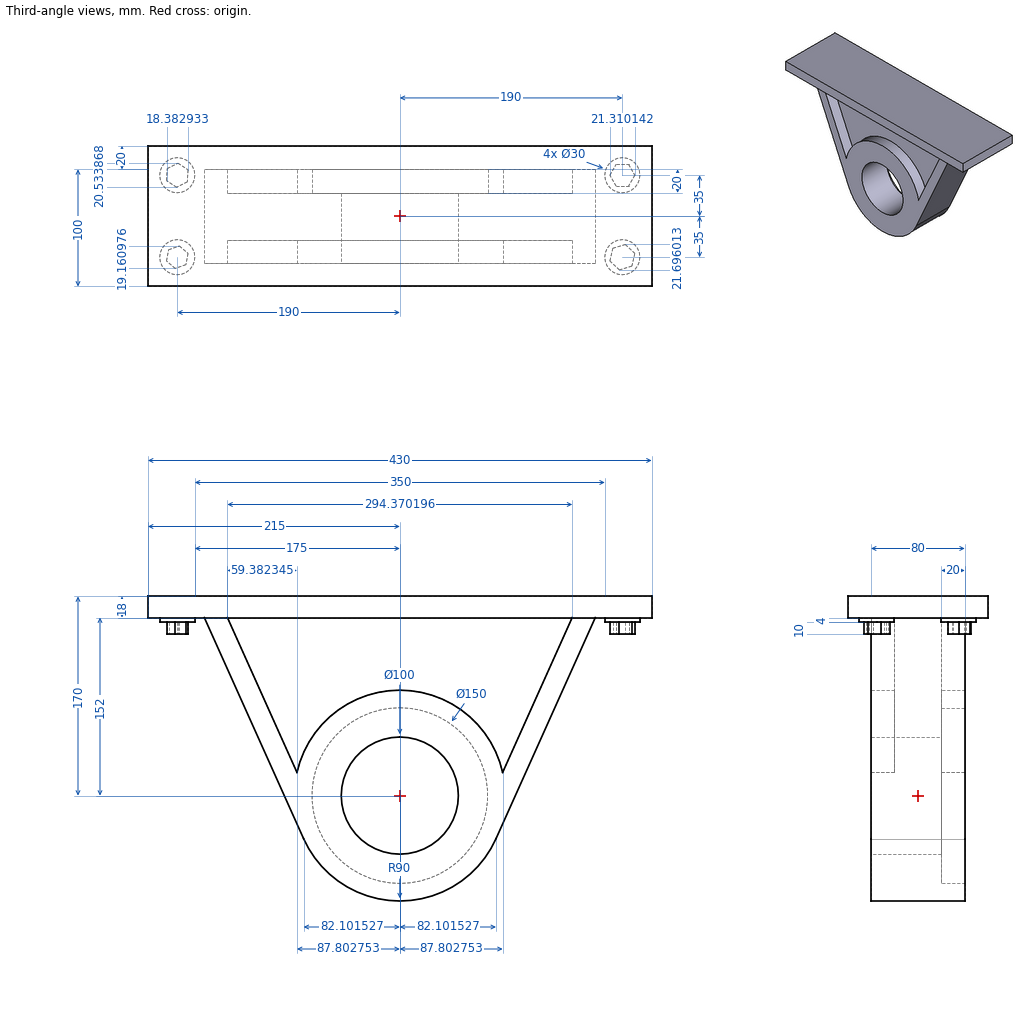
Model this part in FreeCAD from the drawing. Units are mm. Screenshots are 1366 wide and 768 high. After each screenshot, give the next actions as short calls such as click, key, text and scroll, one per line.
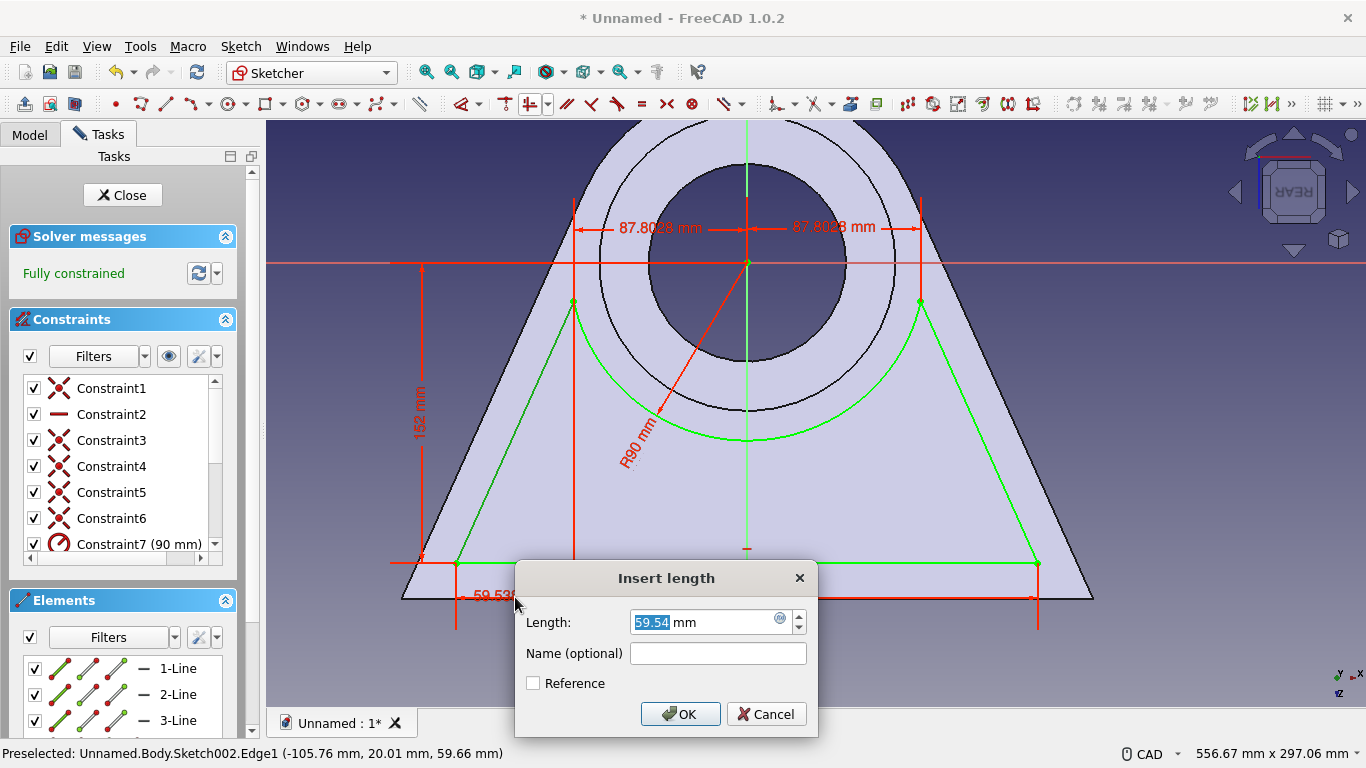
text(59.382345)
key(Return)
key(Escape)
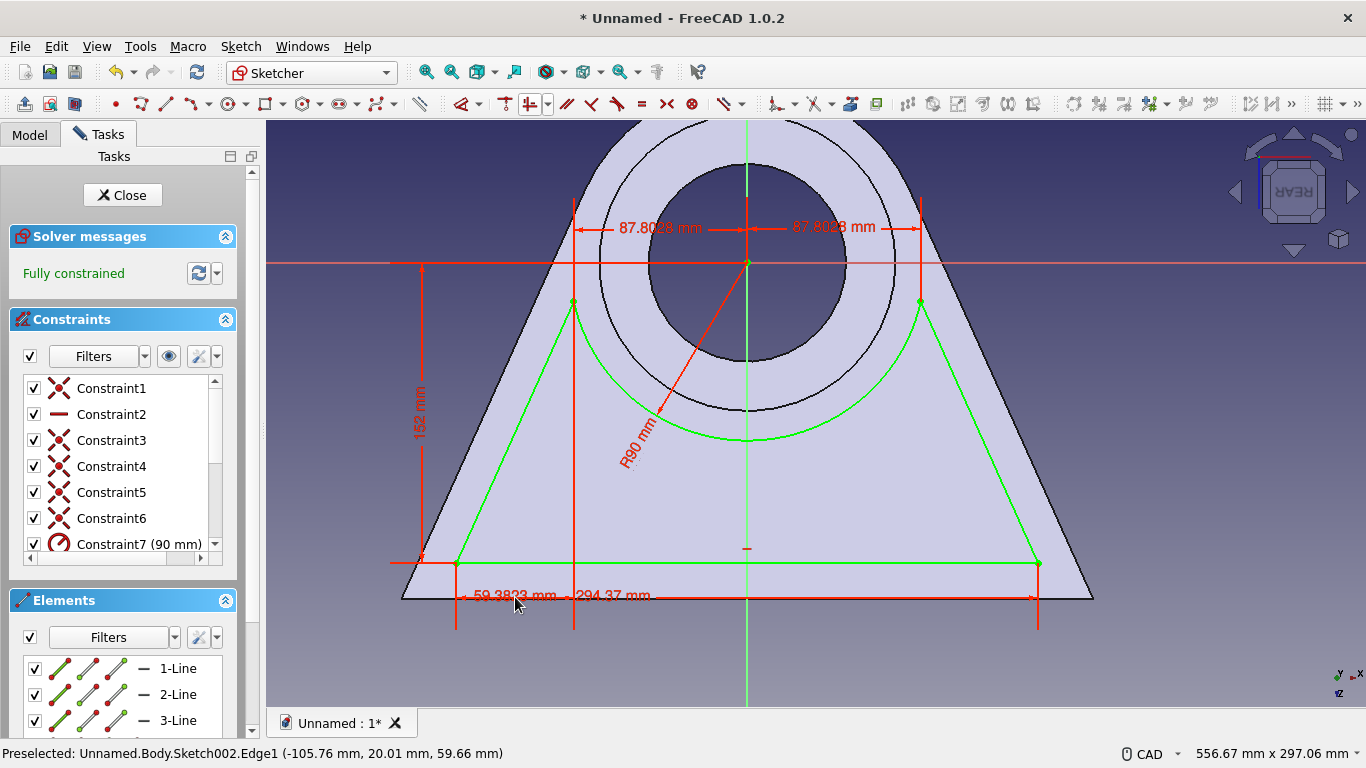
click(123, 195)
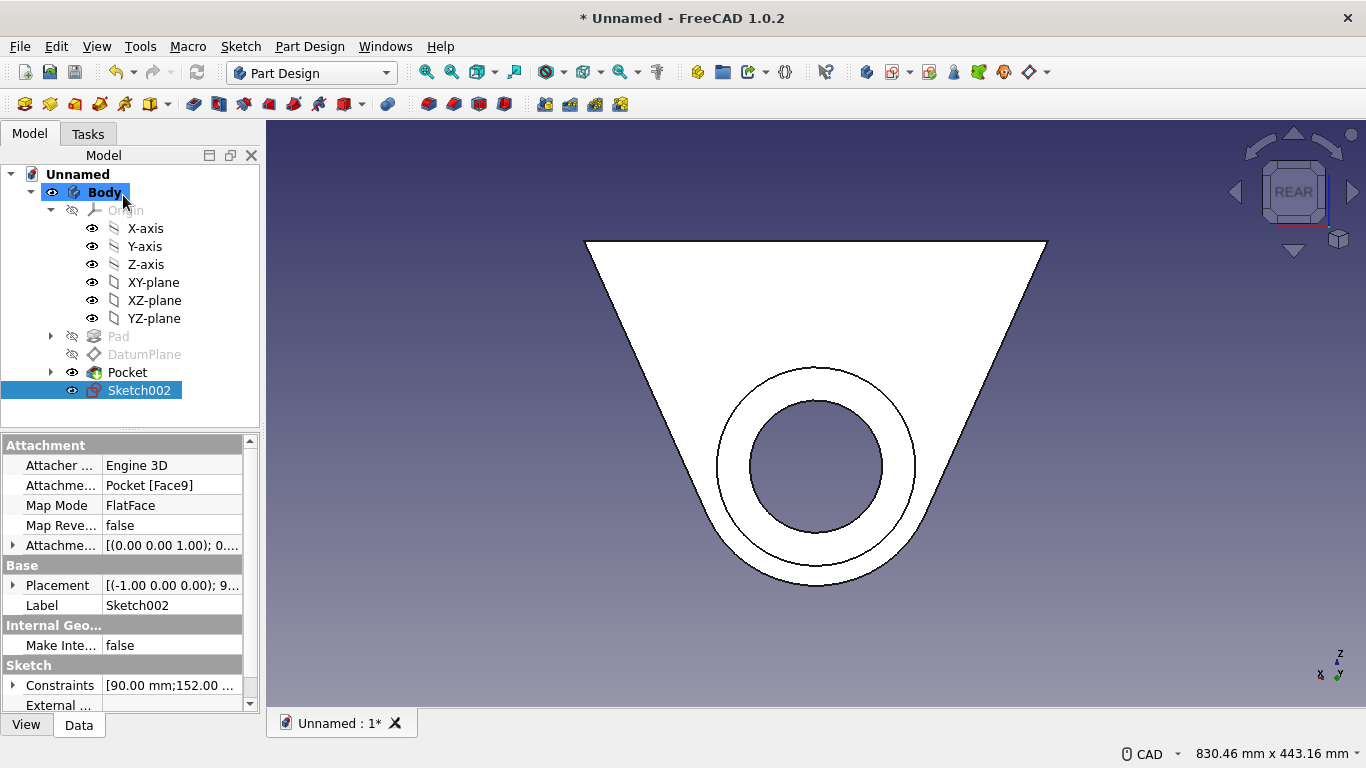
click(194, 104)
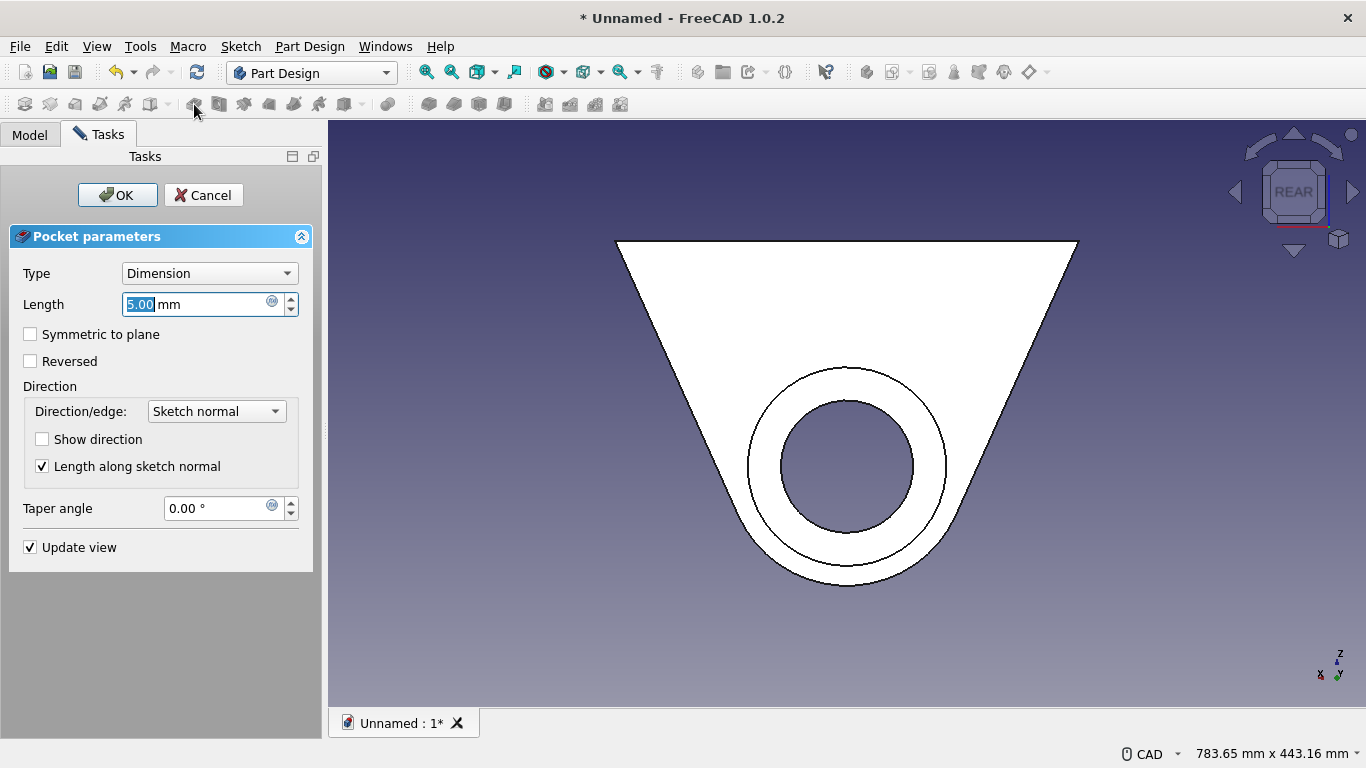
text(20)
key(Tab)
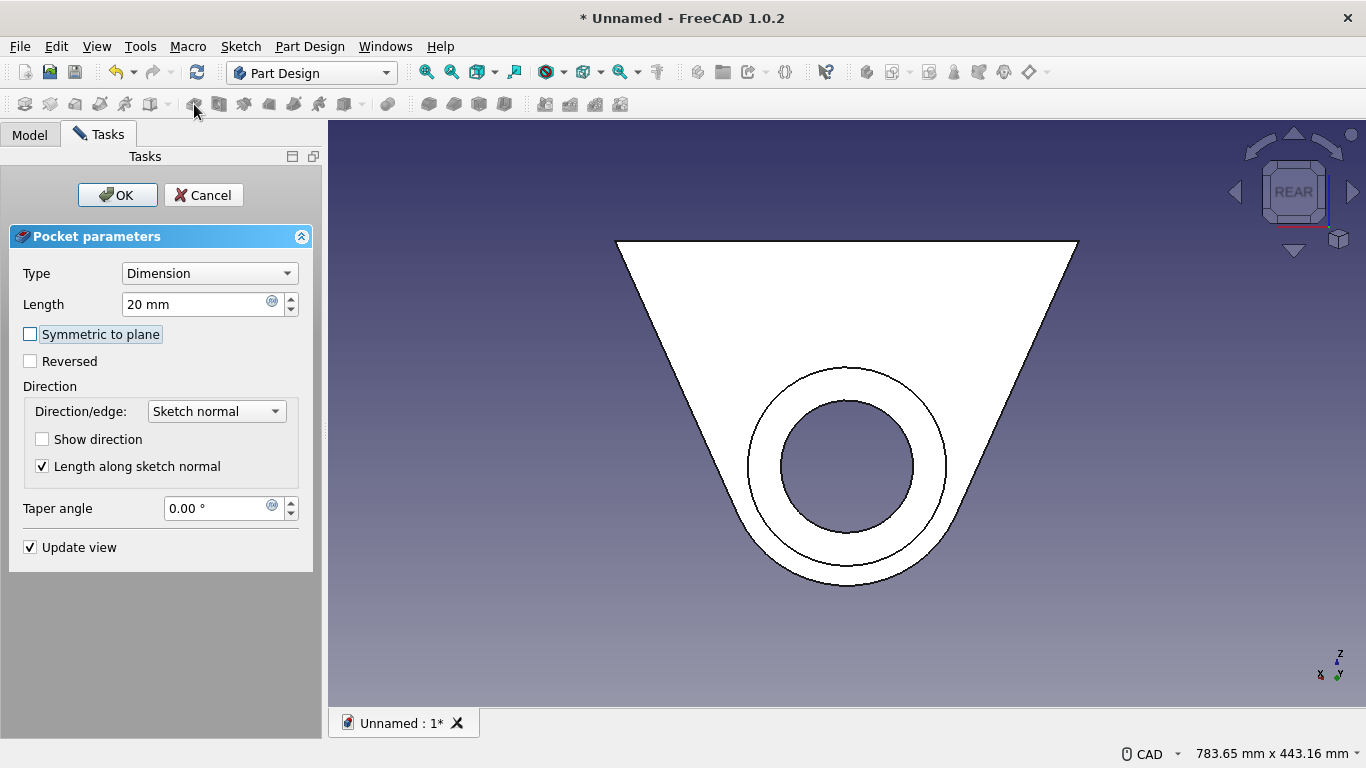
click(31, 361)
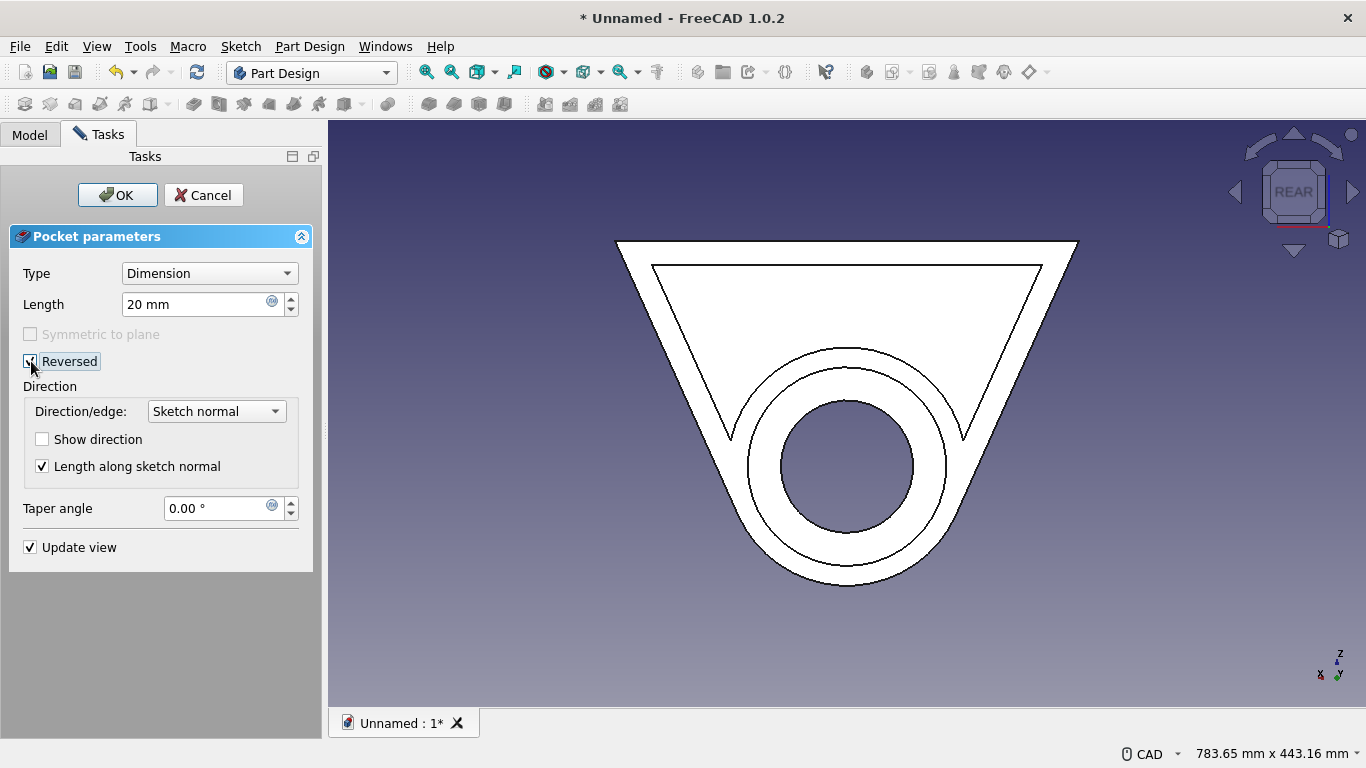
click(118, 195)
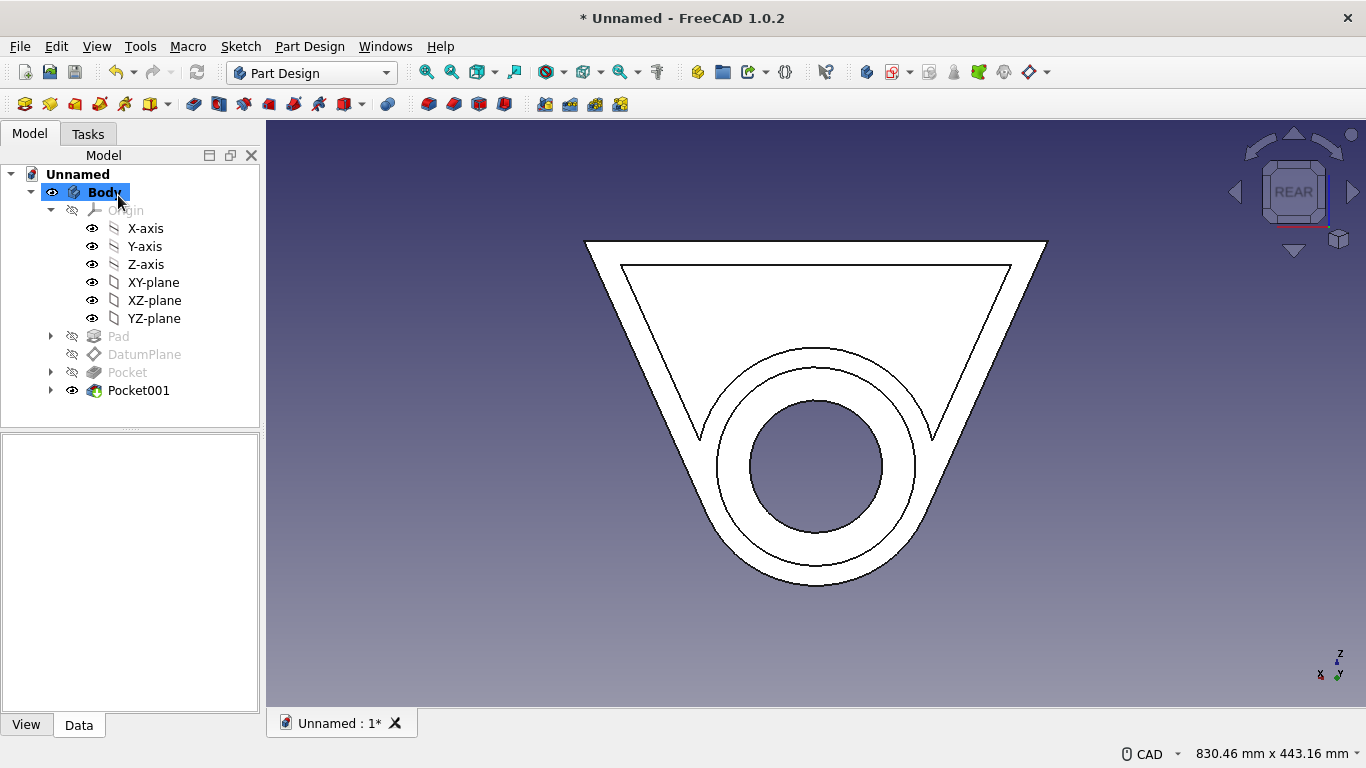
click(117, 390)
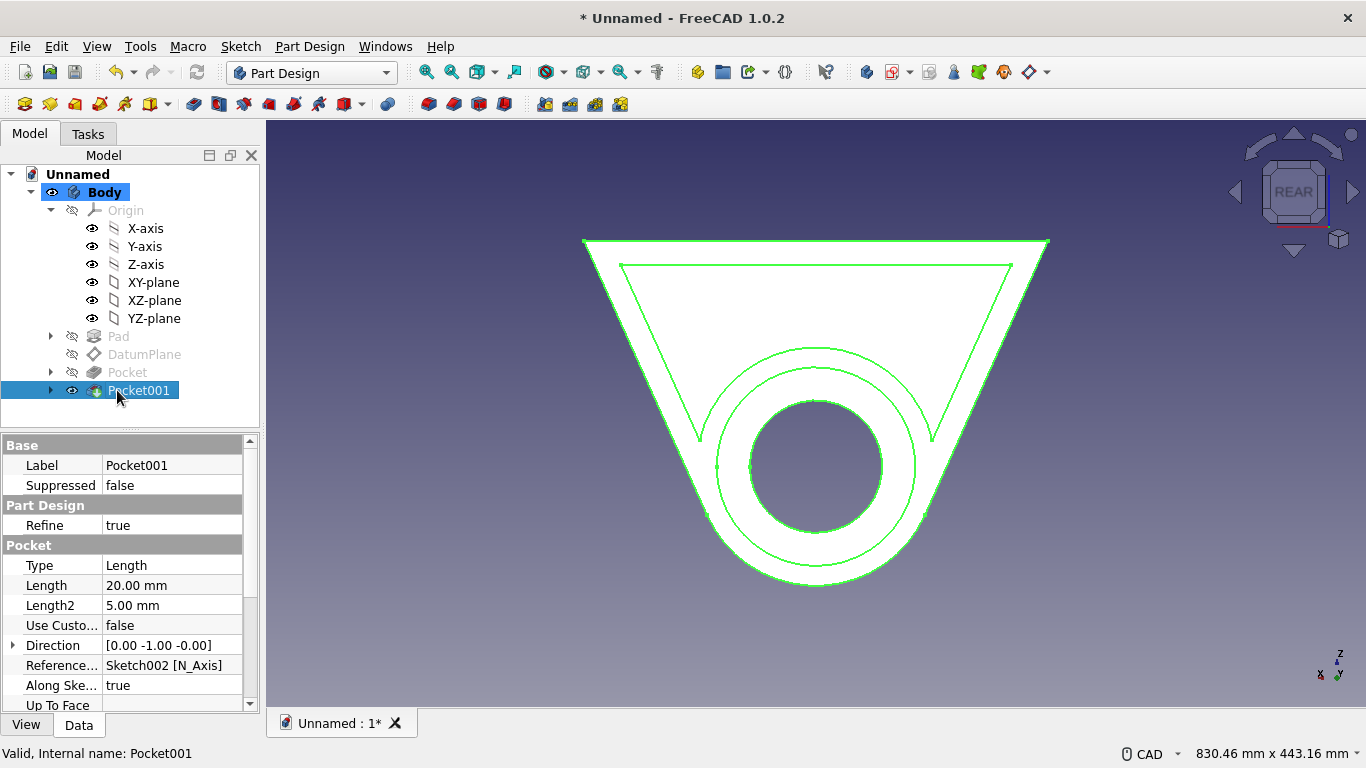
click(545, 104)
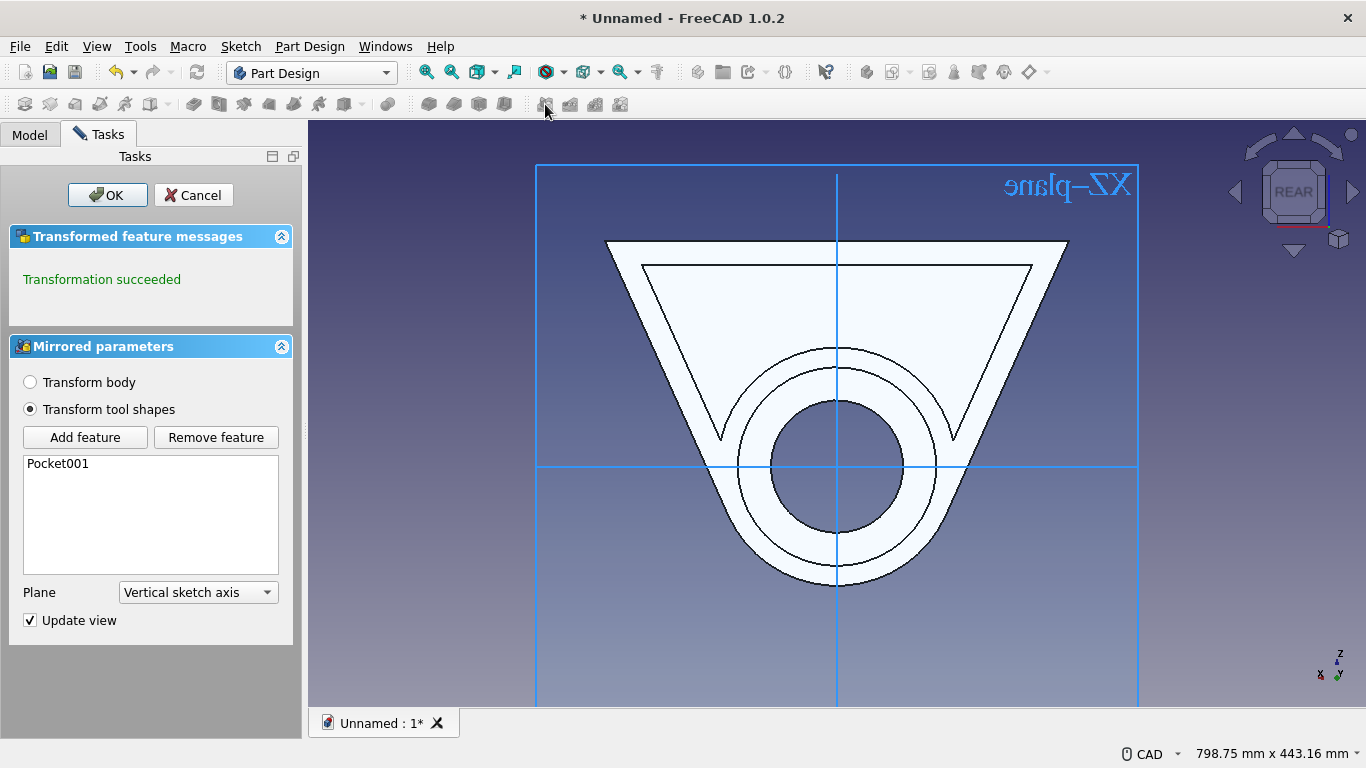
click(199, 592)